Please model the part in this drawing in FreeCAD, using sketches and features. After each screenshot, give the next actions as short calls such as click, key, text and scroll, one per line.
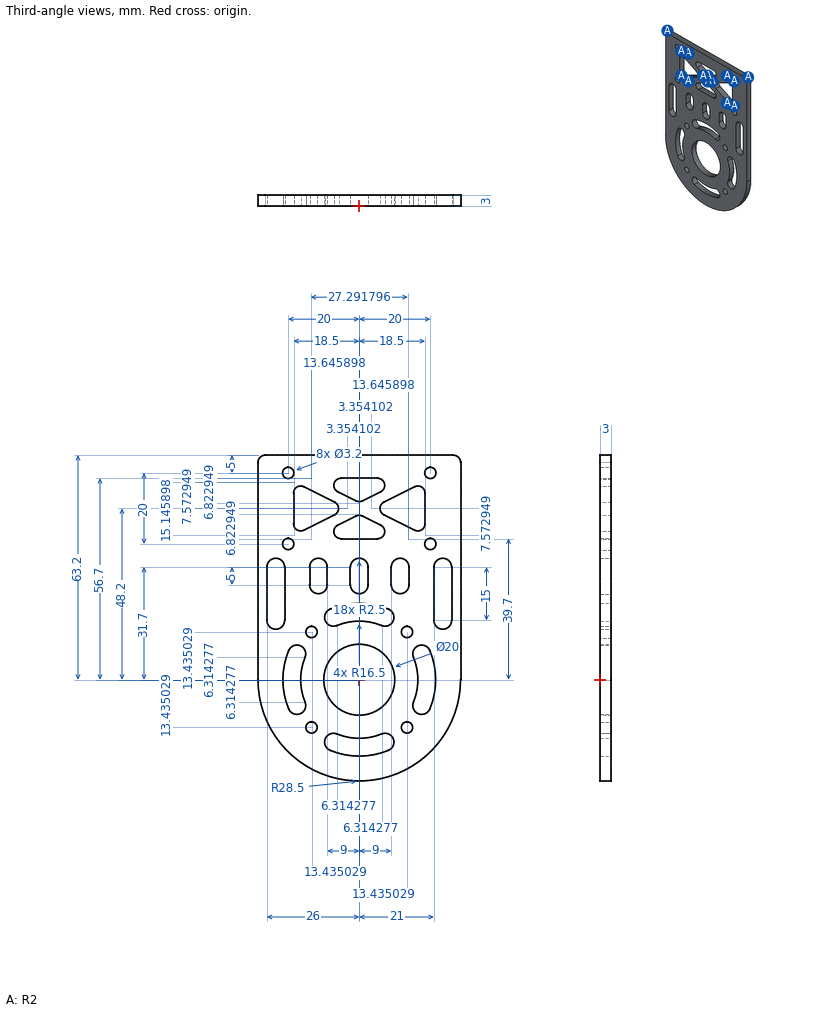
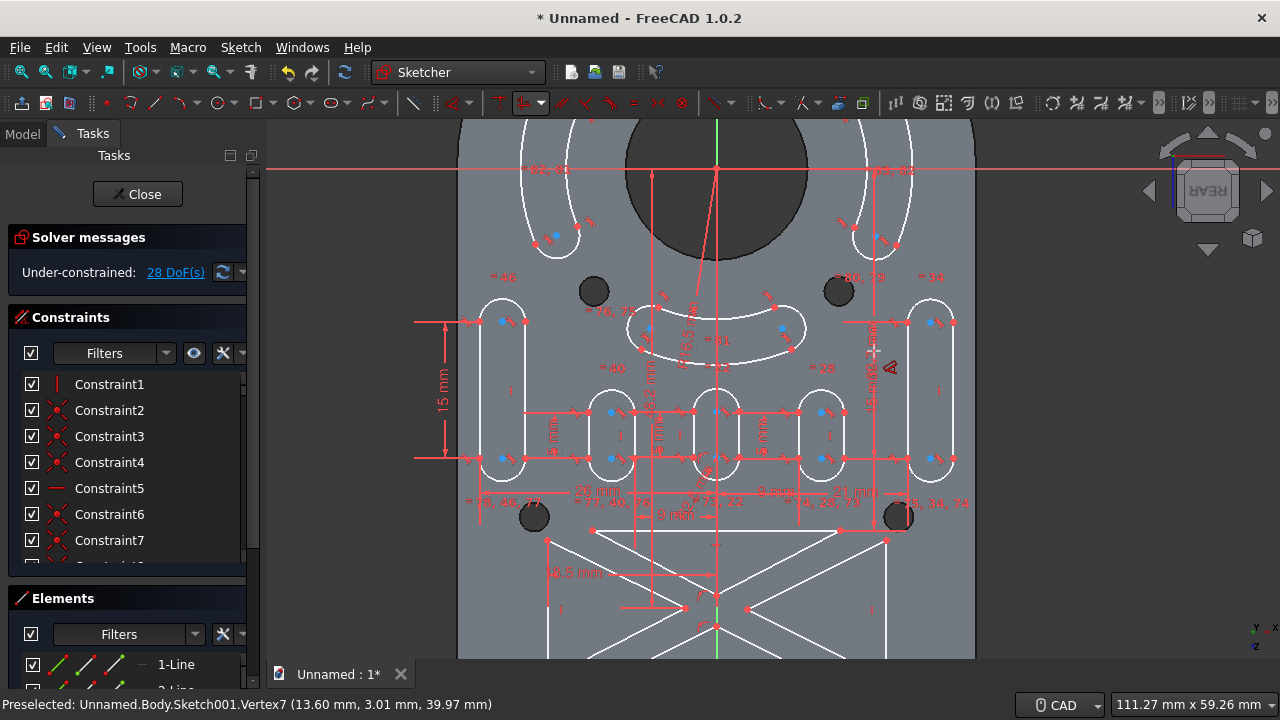
click(886, 540)
click(861, 574)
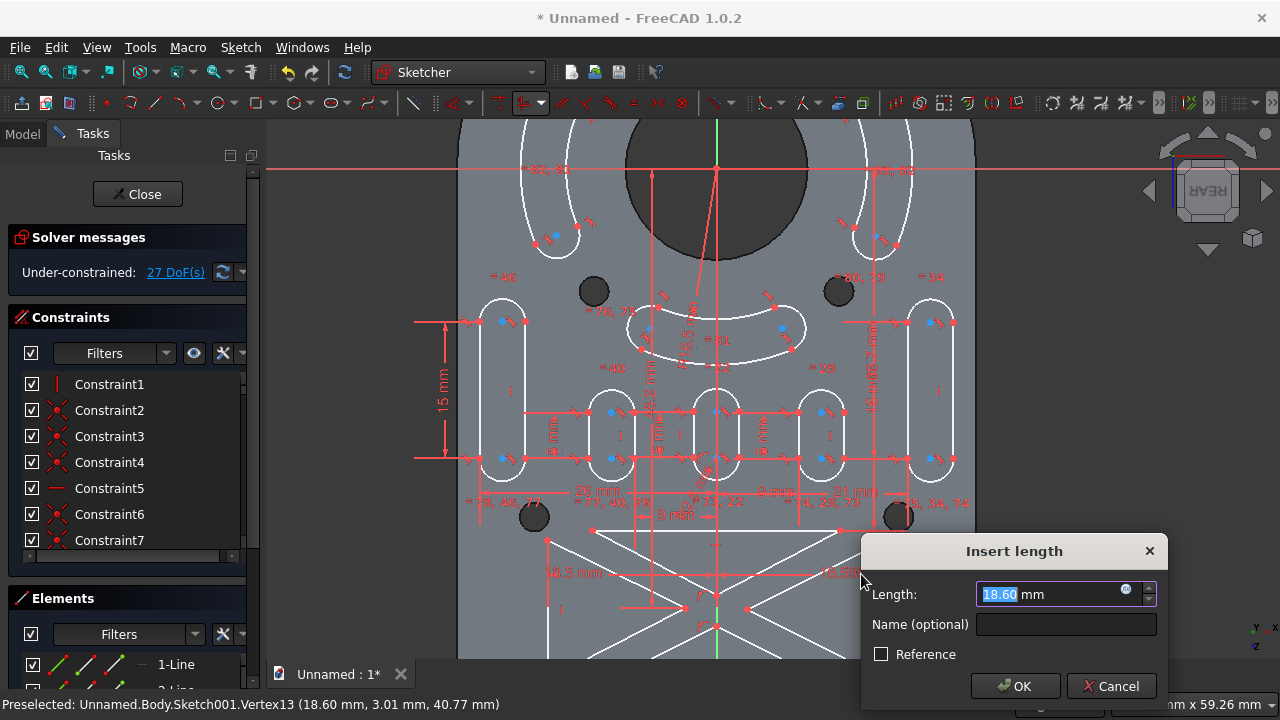
text(18.5)
key(Return)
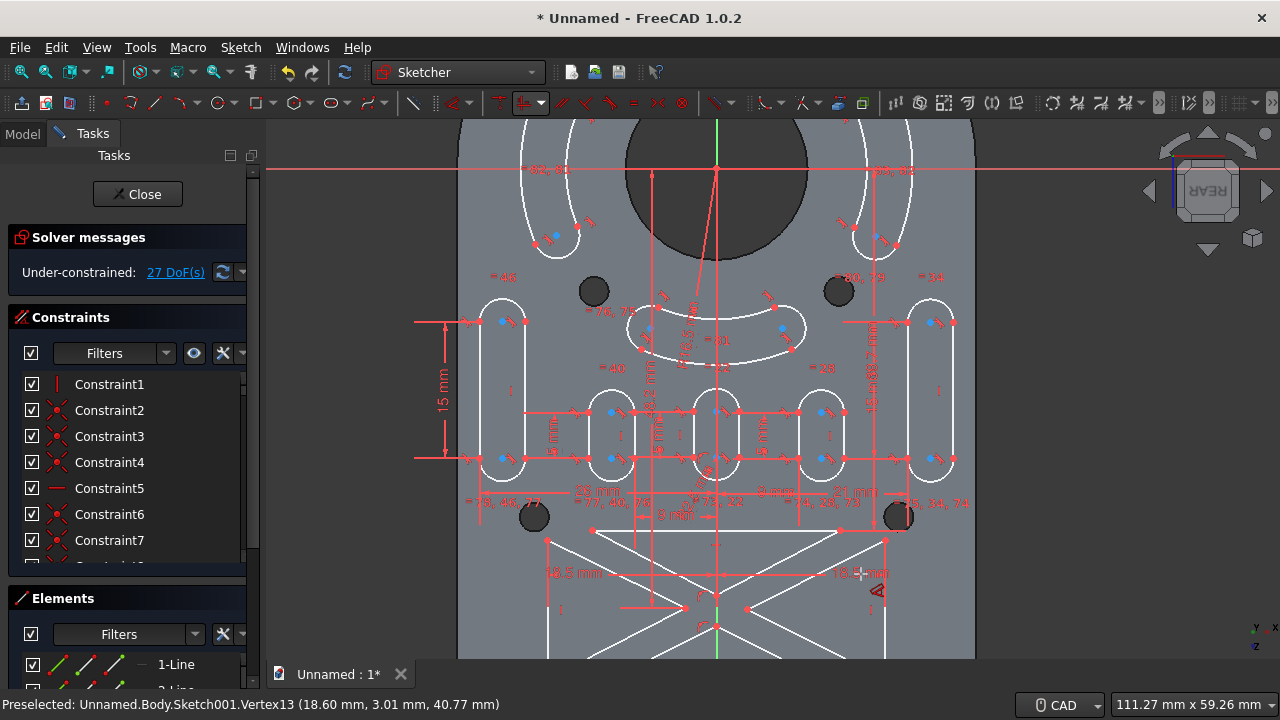
click(748, 610)
click(782, 389)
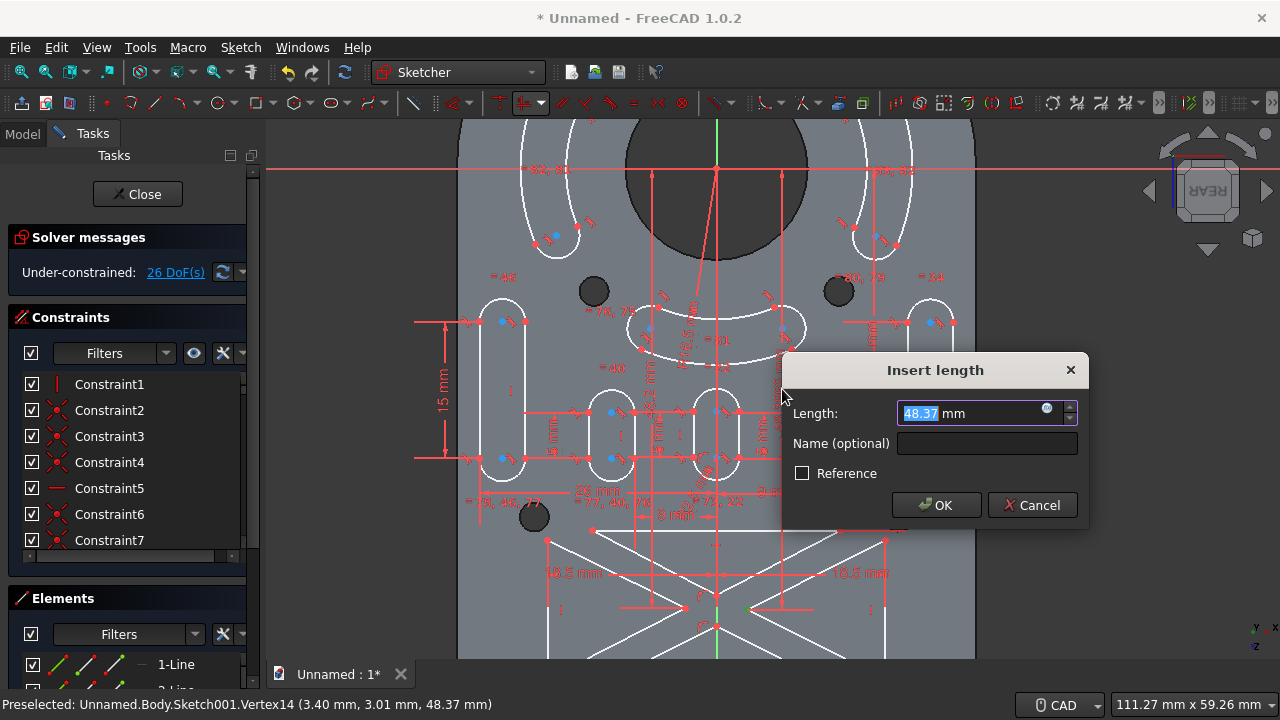
text(48.2)
key(Return)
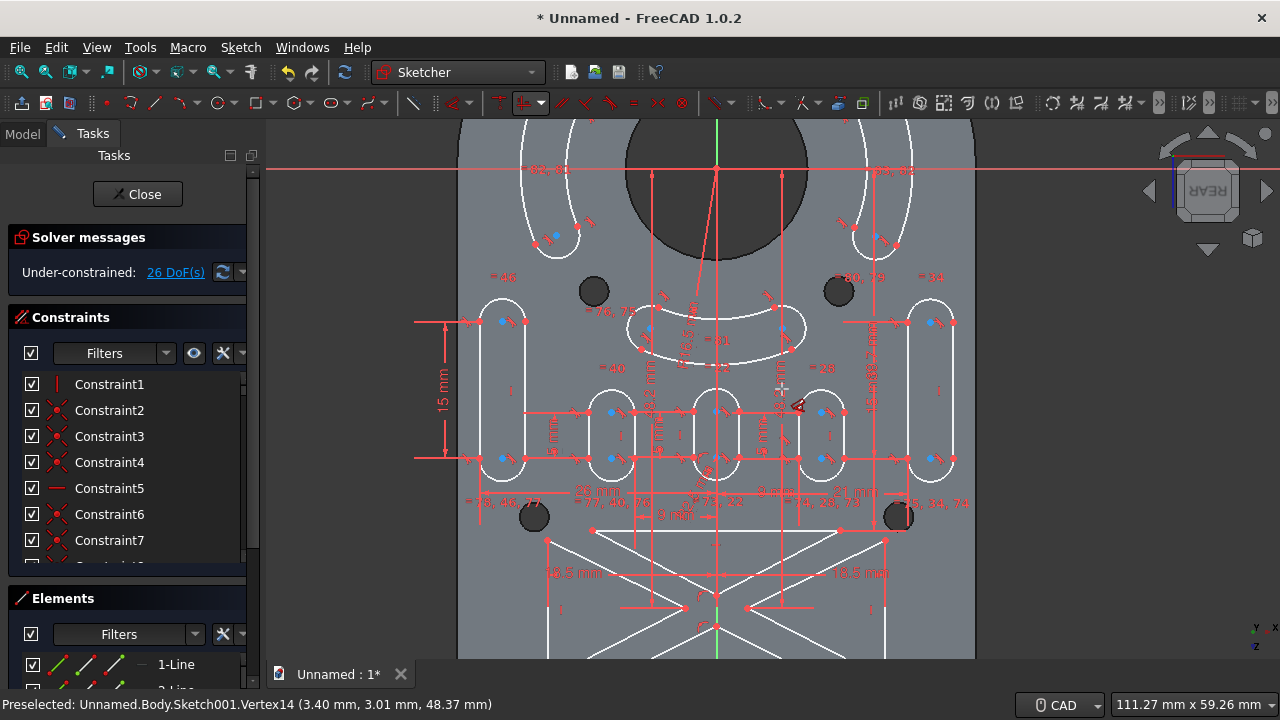
scroll(695, 438, down, 4)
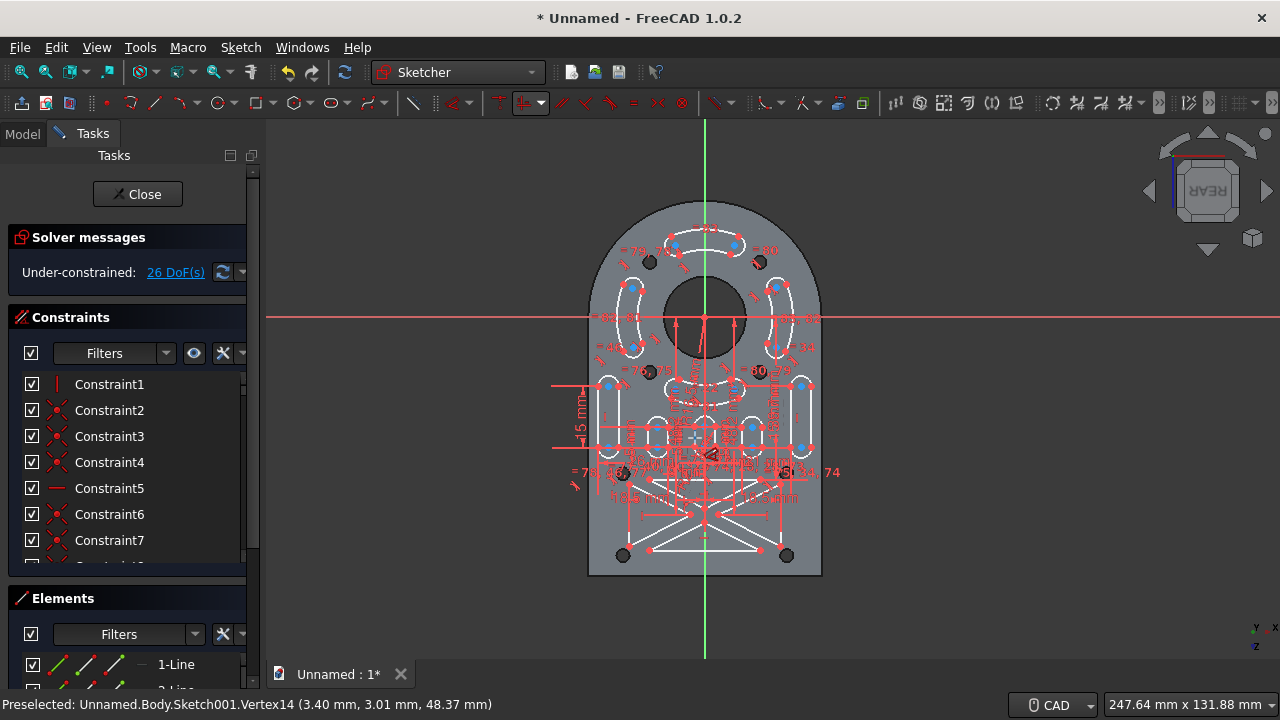
click(649, 551)
click(739, 352)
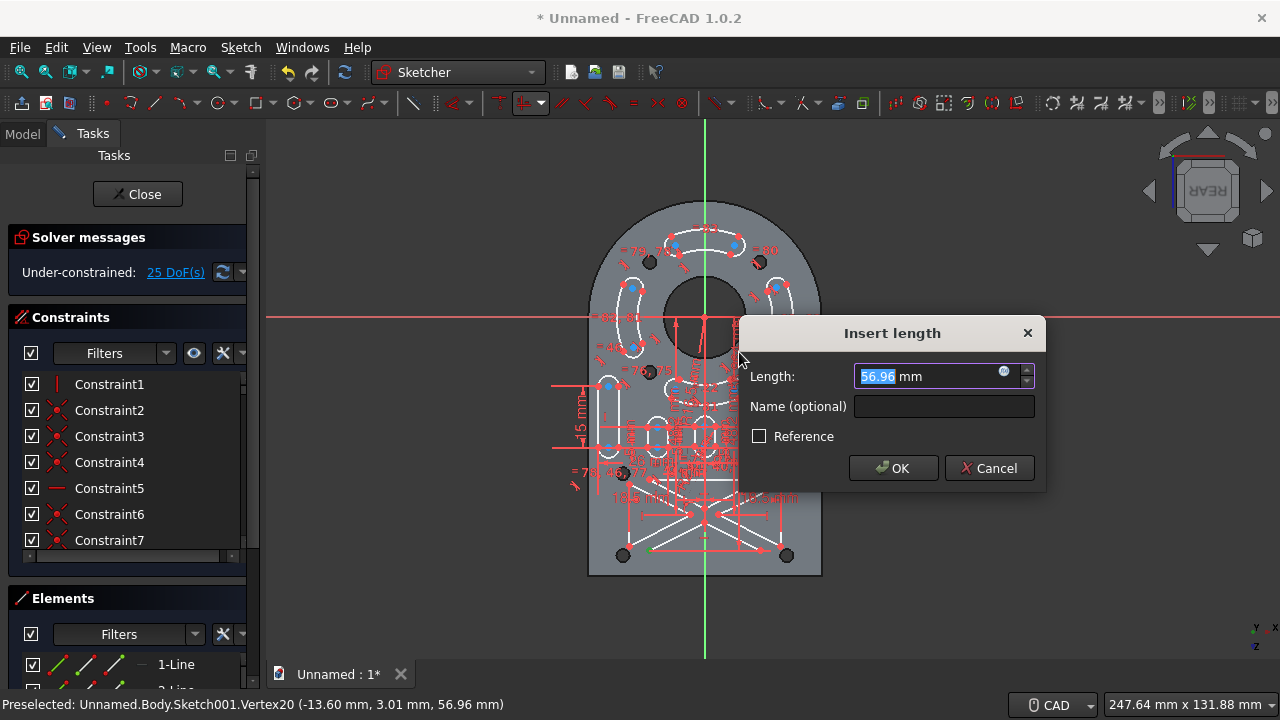
text(56.7)
key(Return)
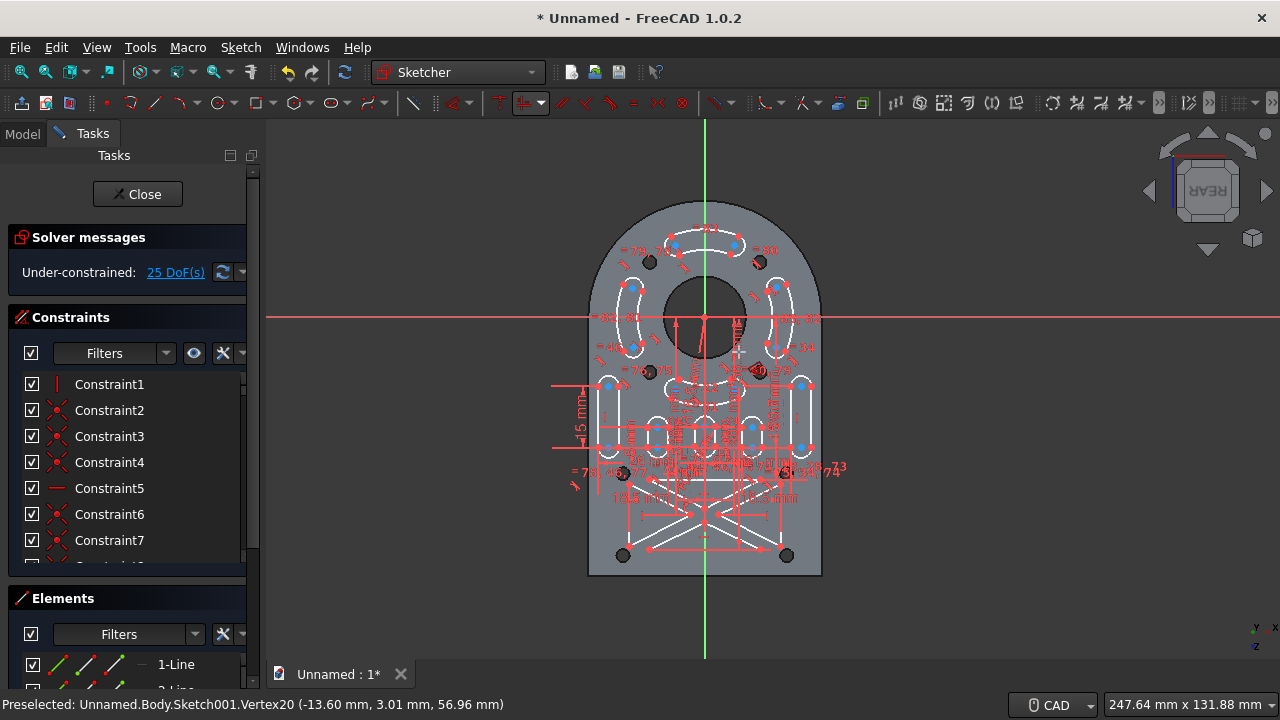
click(695, 447)
click(661, 352)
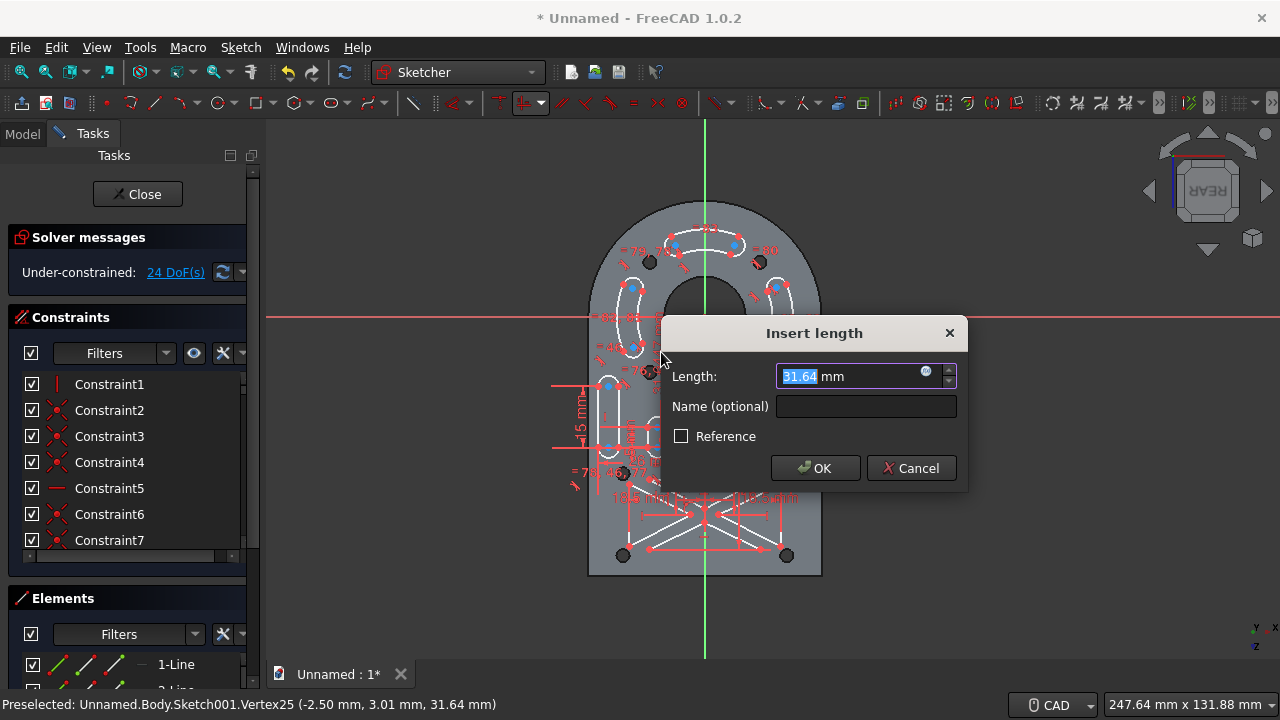
text(31.7)
key(Return)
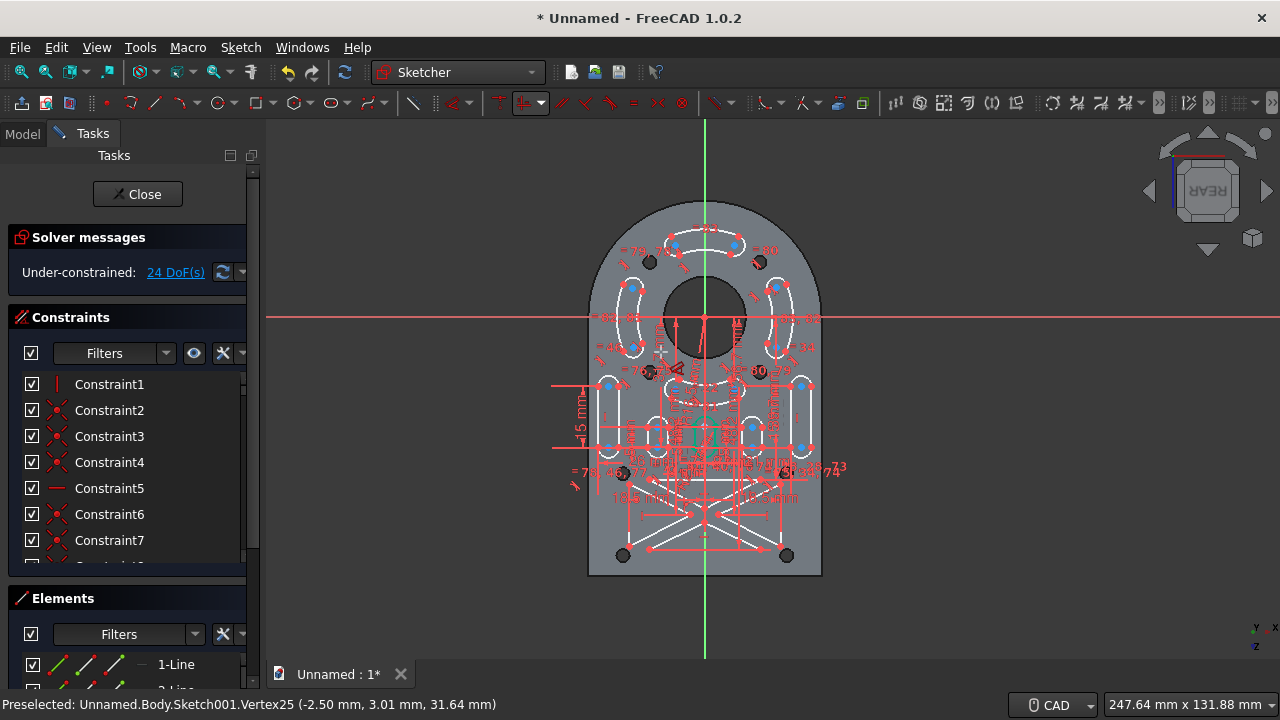
click(742, 448)
click(824, 353)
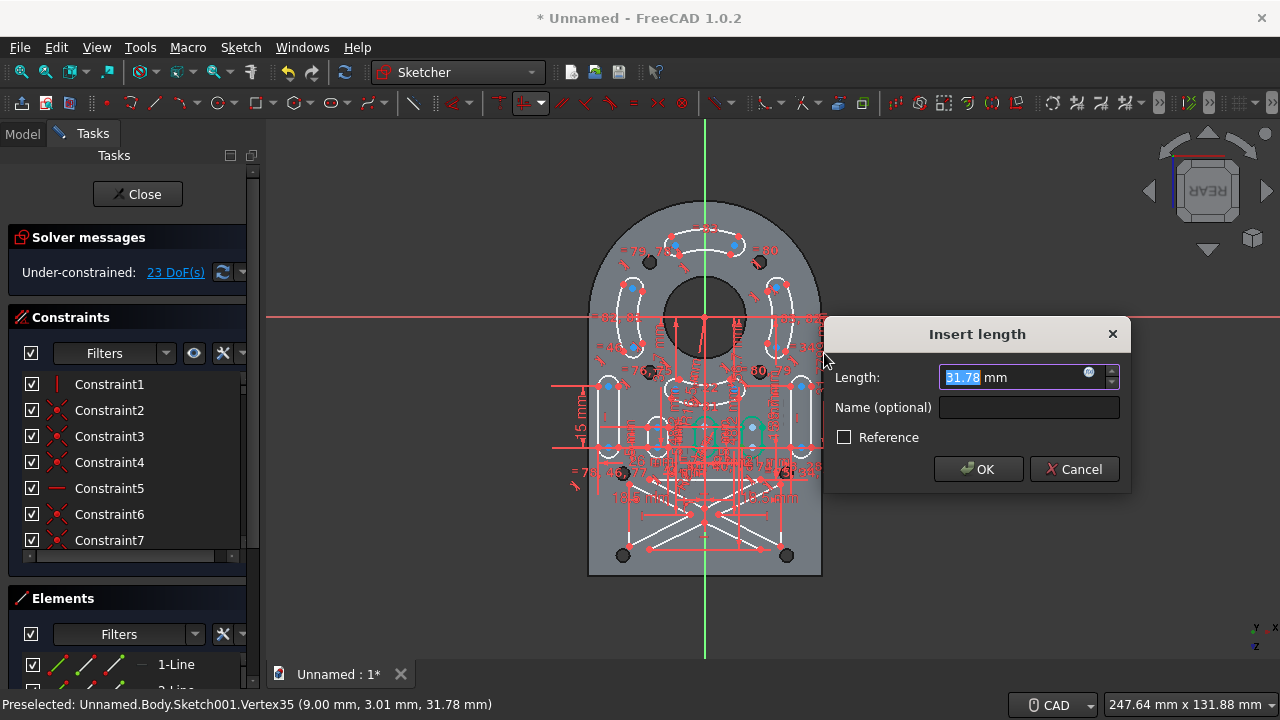
text(31.7)
key(Return)